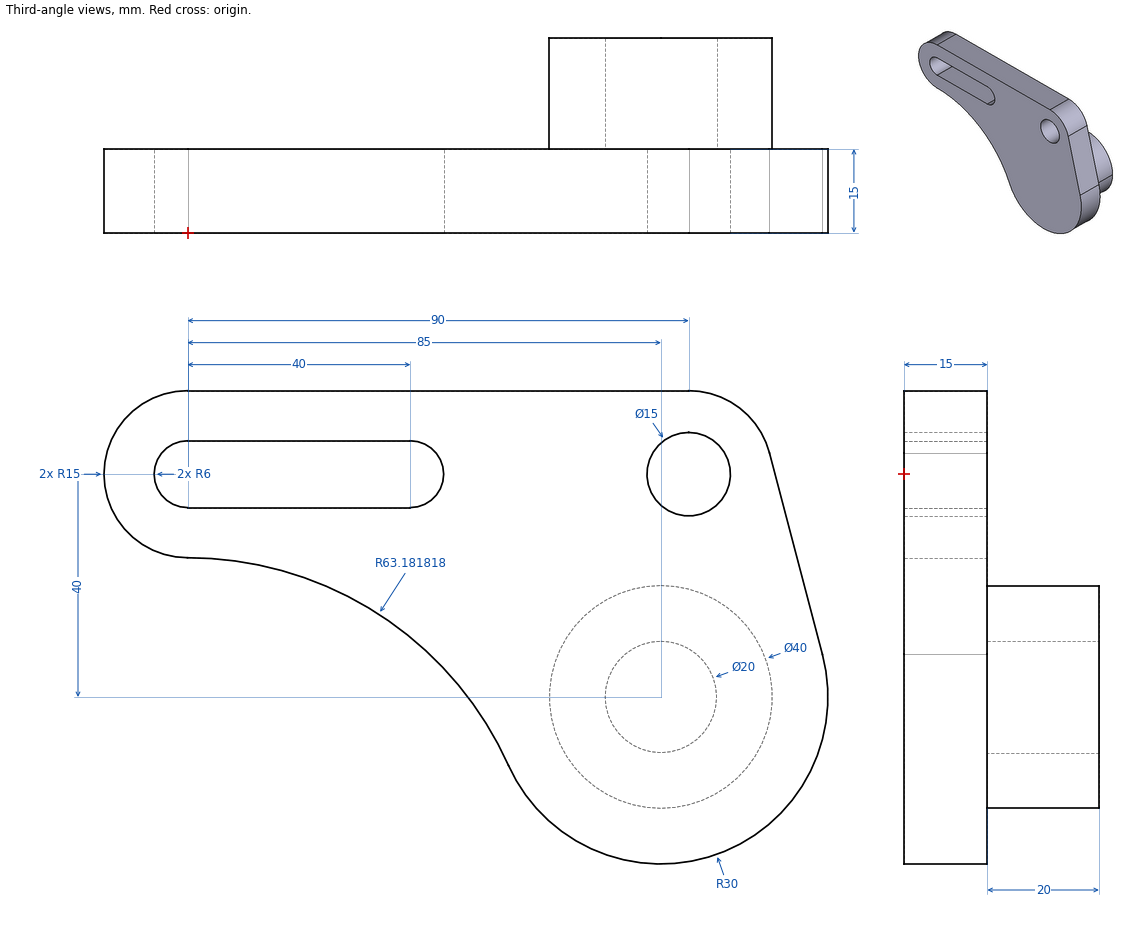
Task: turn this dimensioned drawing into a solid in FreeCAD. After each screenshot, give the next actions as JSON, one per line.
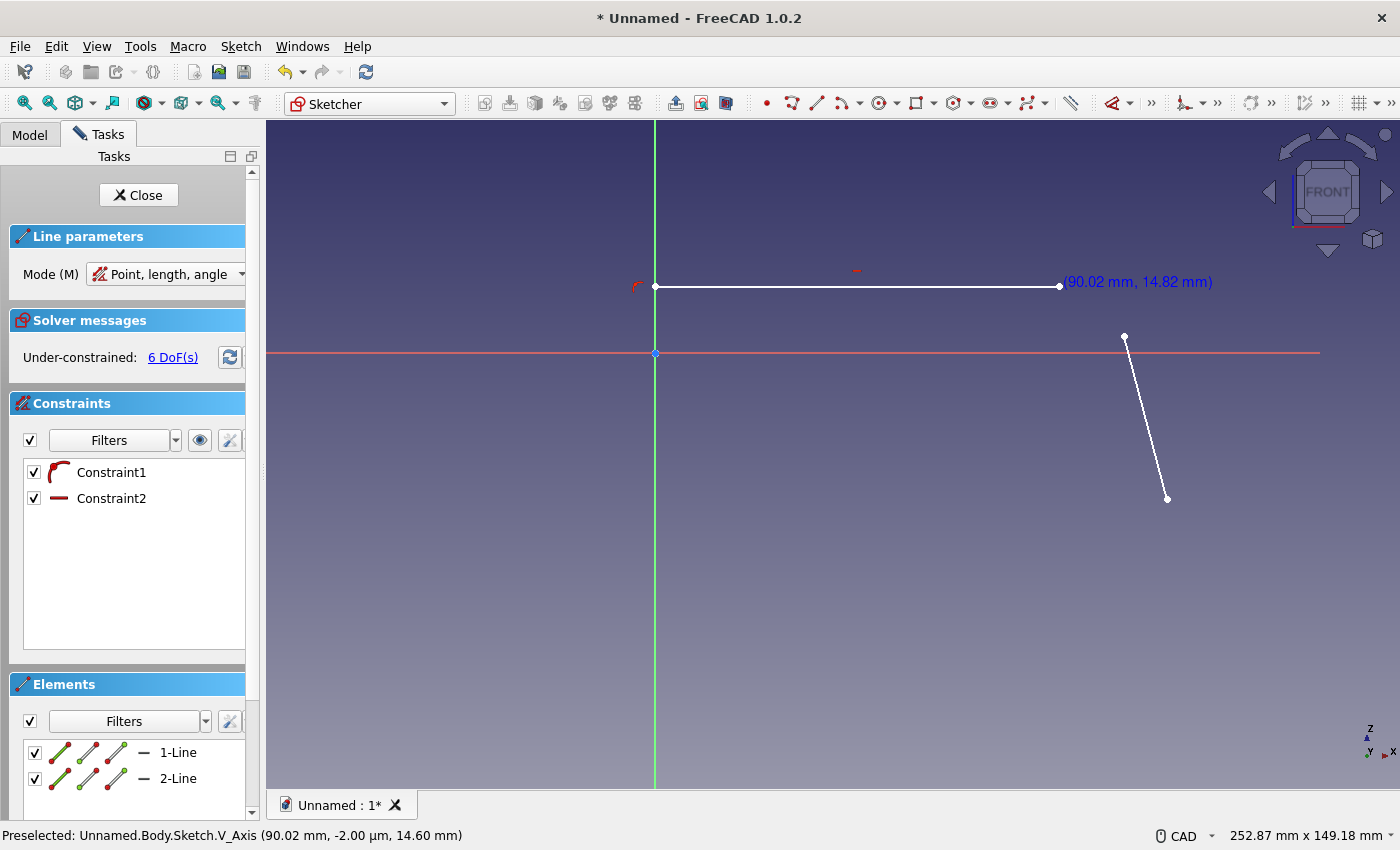
{"action": "left_click", "coordinate": [860, 104]}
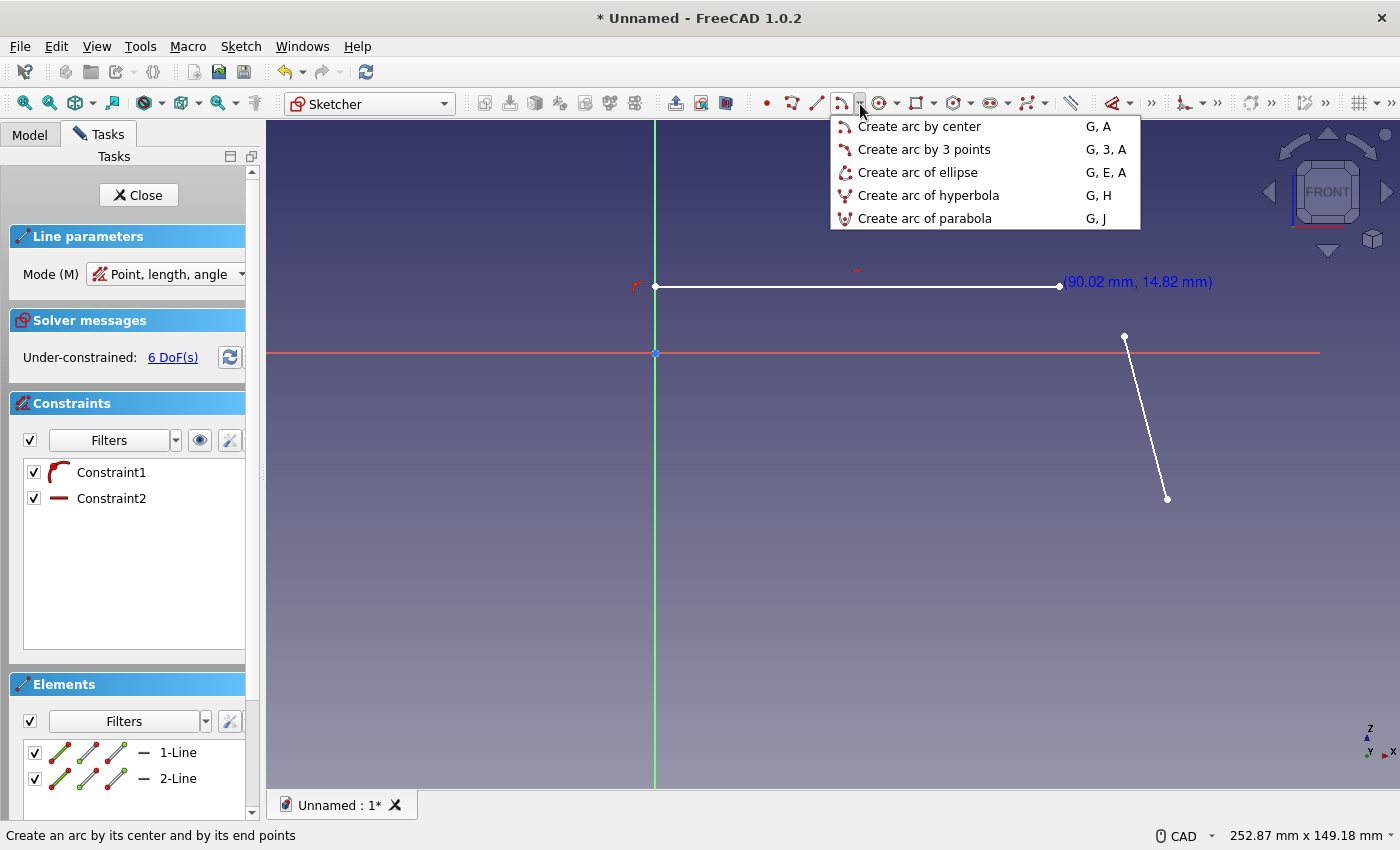
{"action": "left_click", "coordinate": [986, 150]}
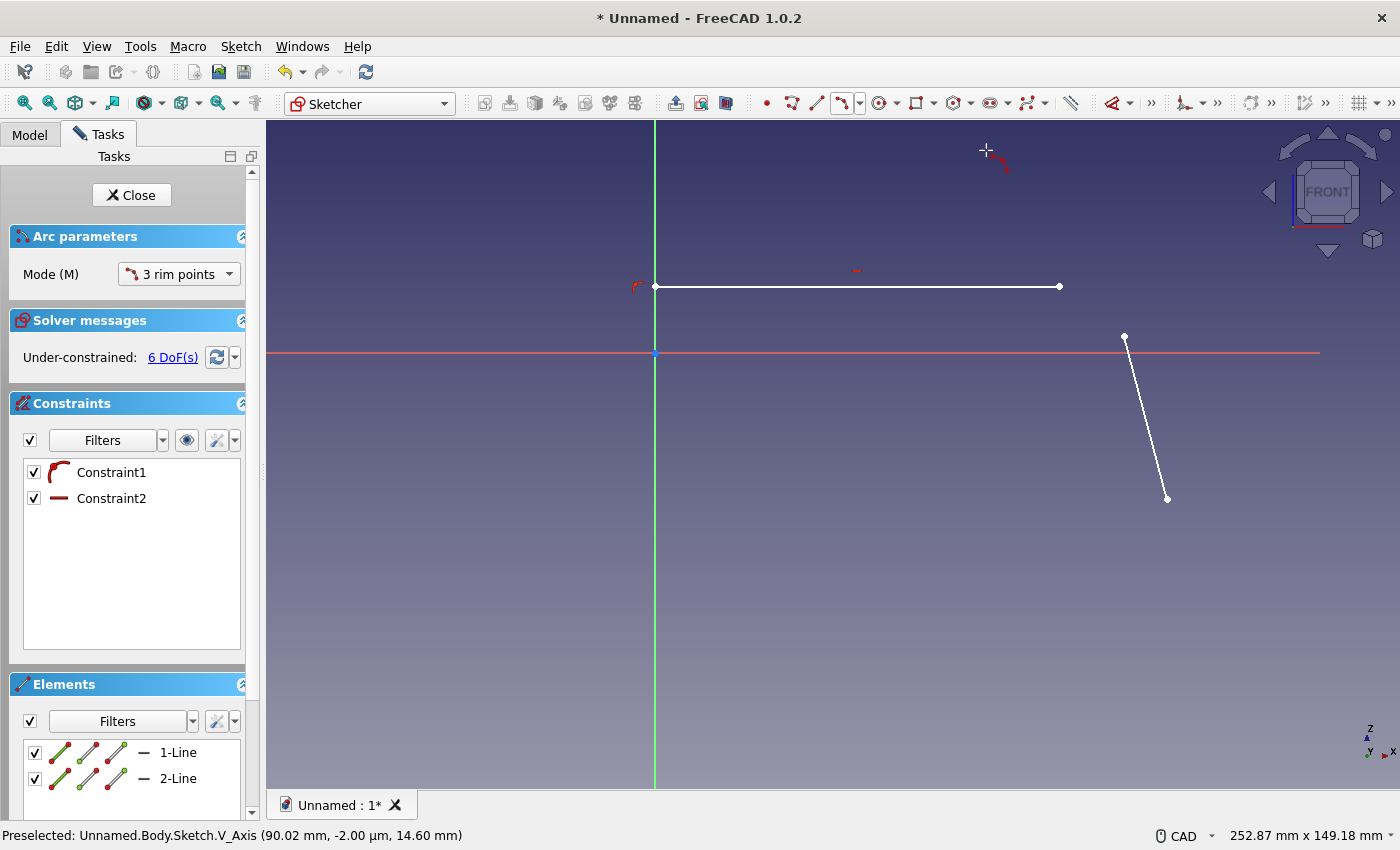
{"action": "left_click", "coordinate": [1167, 500]}
{"action": "left_click", "coordinate": [914, 588]}
{"action": "left_click", "coordinate": [1081, 660]}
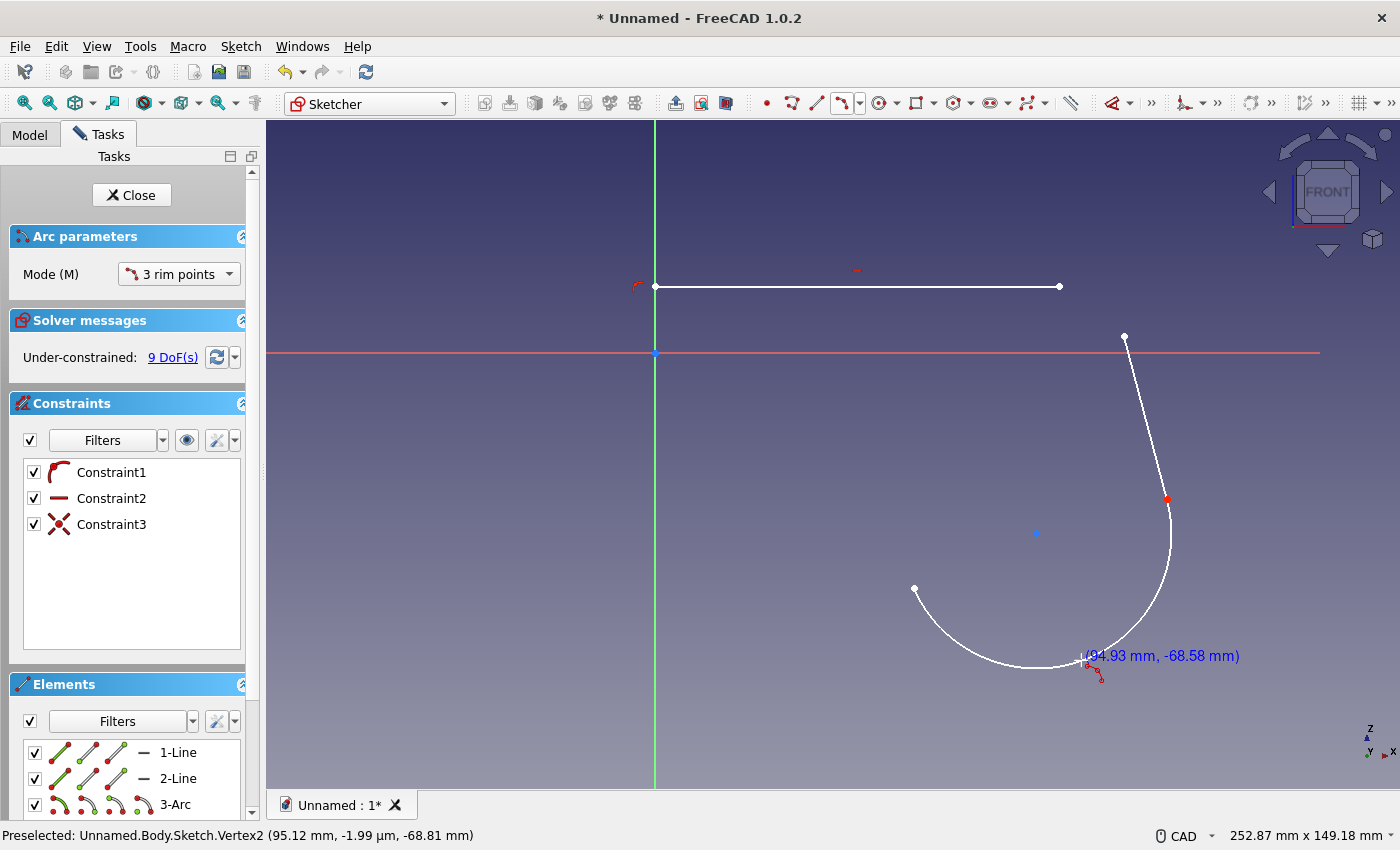
{"action": "left_click", "coordinate": [914, 589]}
{"action": "left_click", "coordinate": [655, 421]}
{"action": "left_click", "coordinate": [809, 466]}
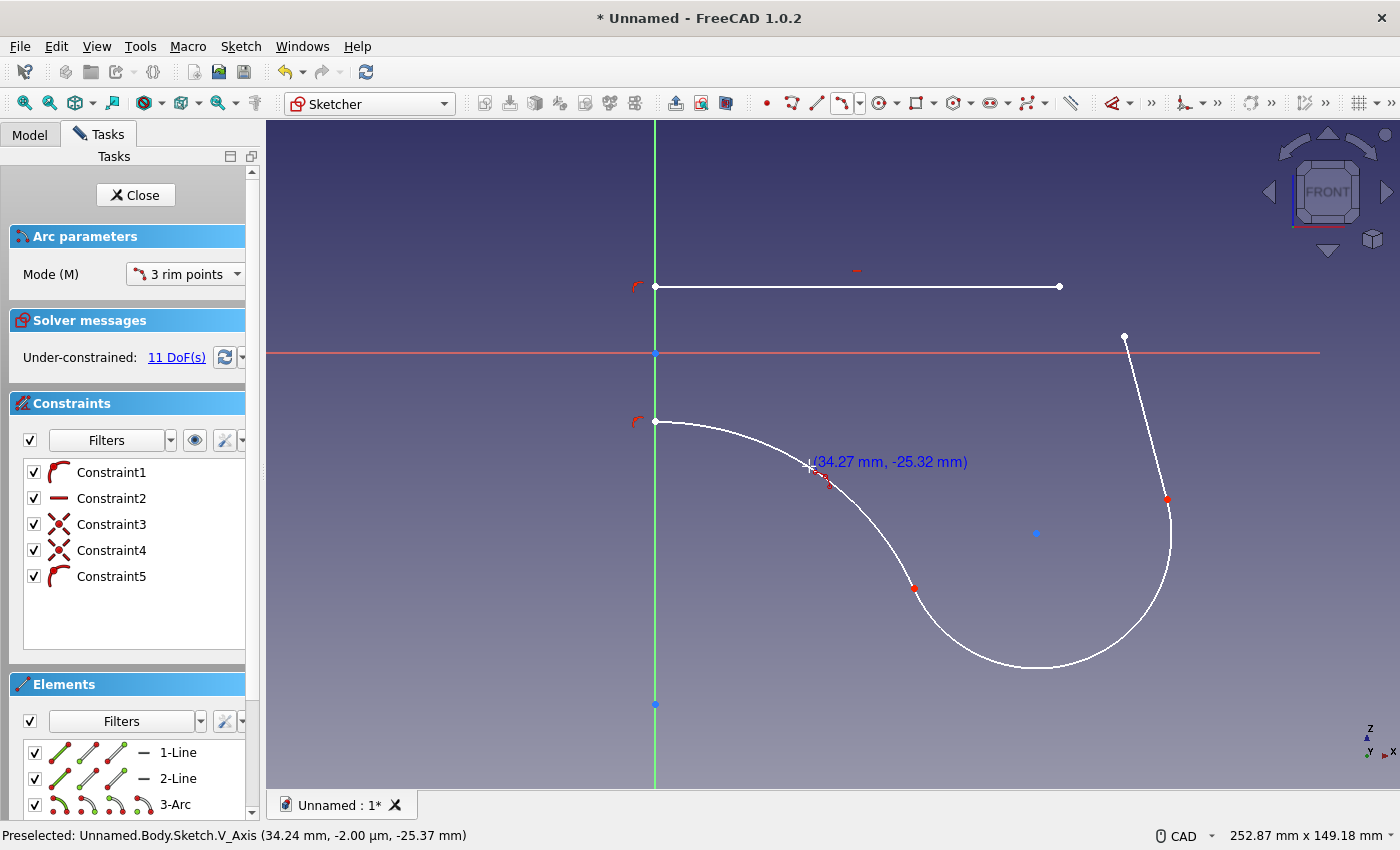
{"action": "left_click", "coordinate": [655, 422]}
{"action": "left_click", "coordinate": [655, 287]}
{"action": "left_click", "coordinate": [591, 333]}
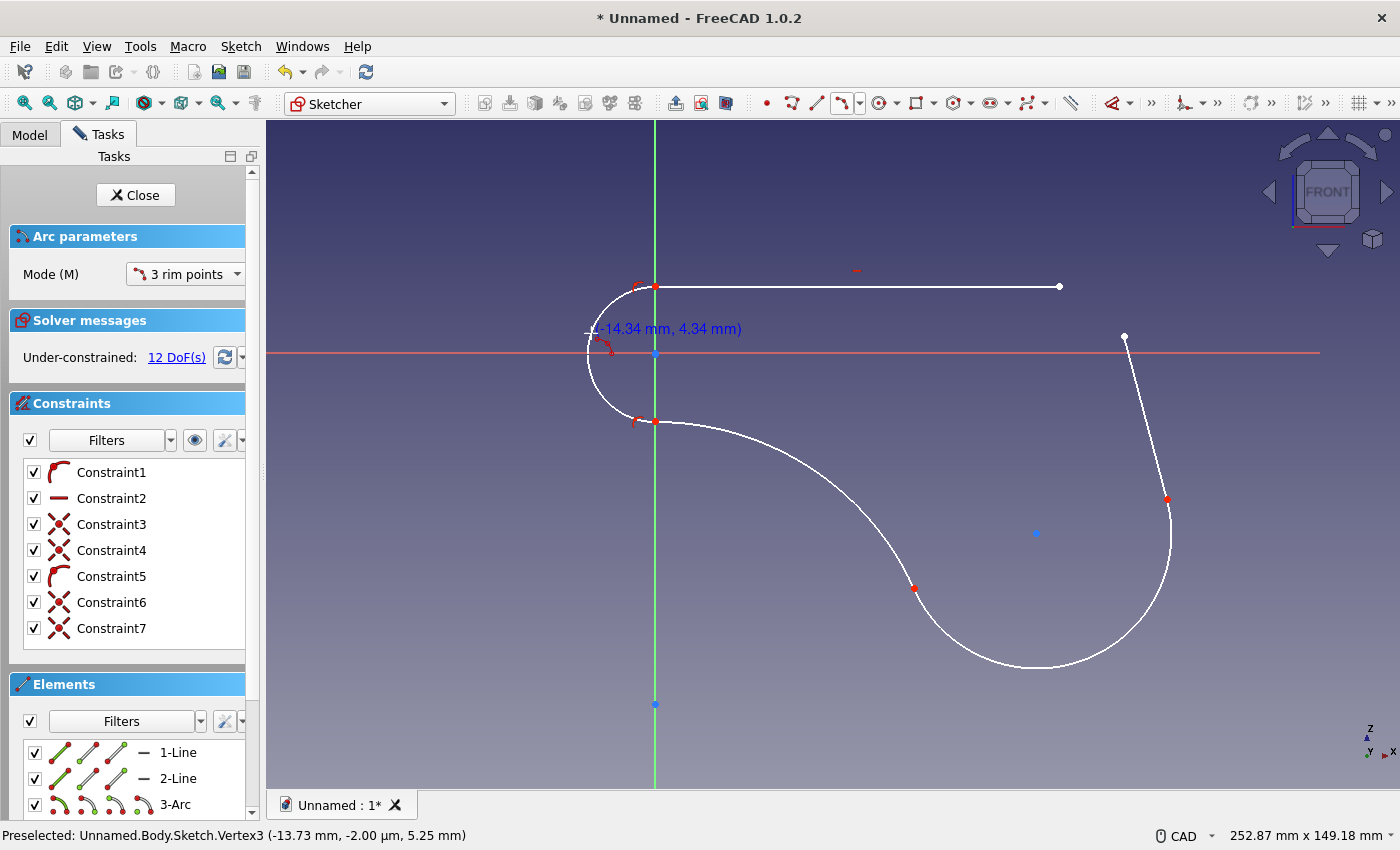
{"action": "left_click", "coordinate": [1059, 287]}
{"action": "left_click", "coordinate": [1124, 337]}
{"action": "left_click", "coordinate": [1100, 300]}
{"action": "key", "text": "Escape"}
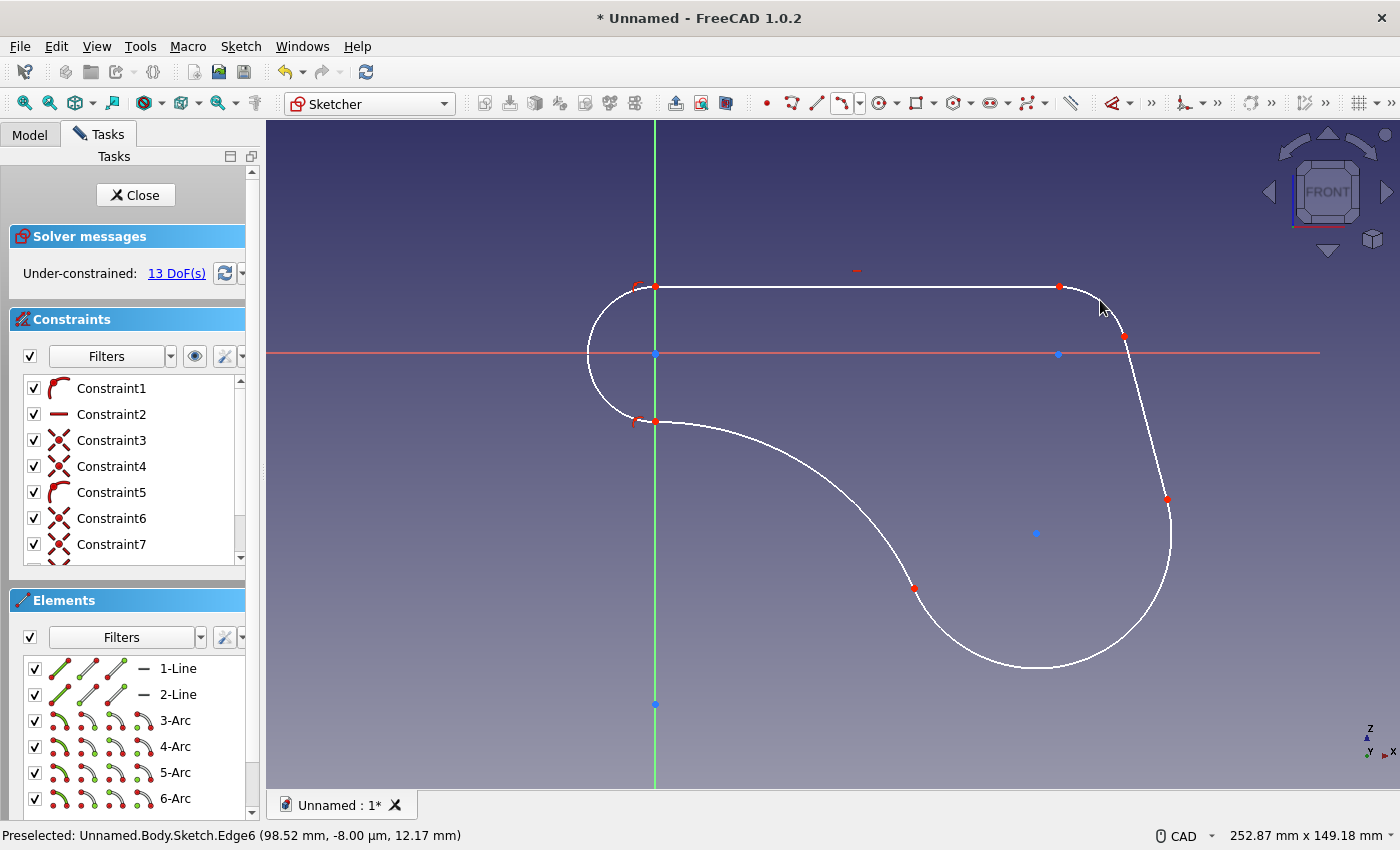
{"action": "left_click", "coordinate": [1137, 386]}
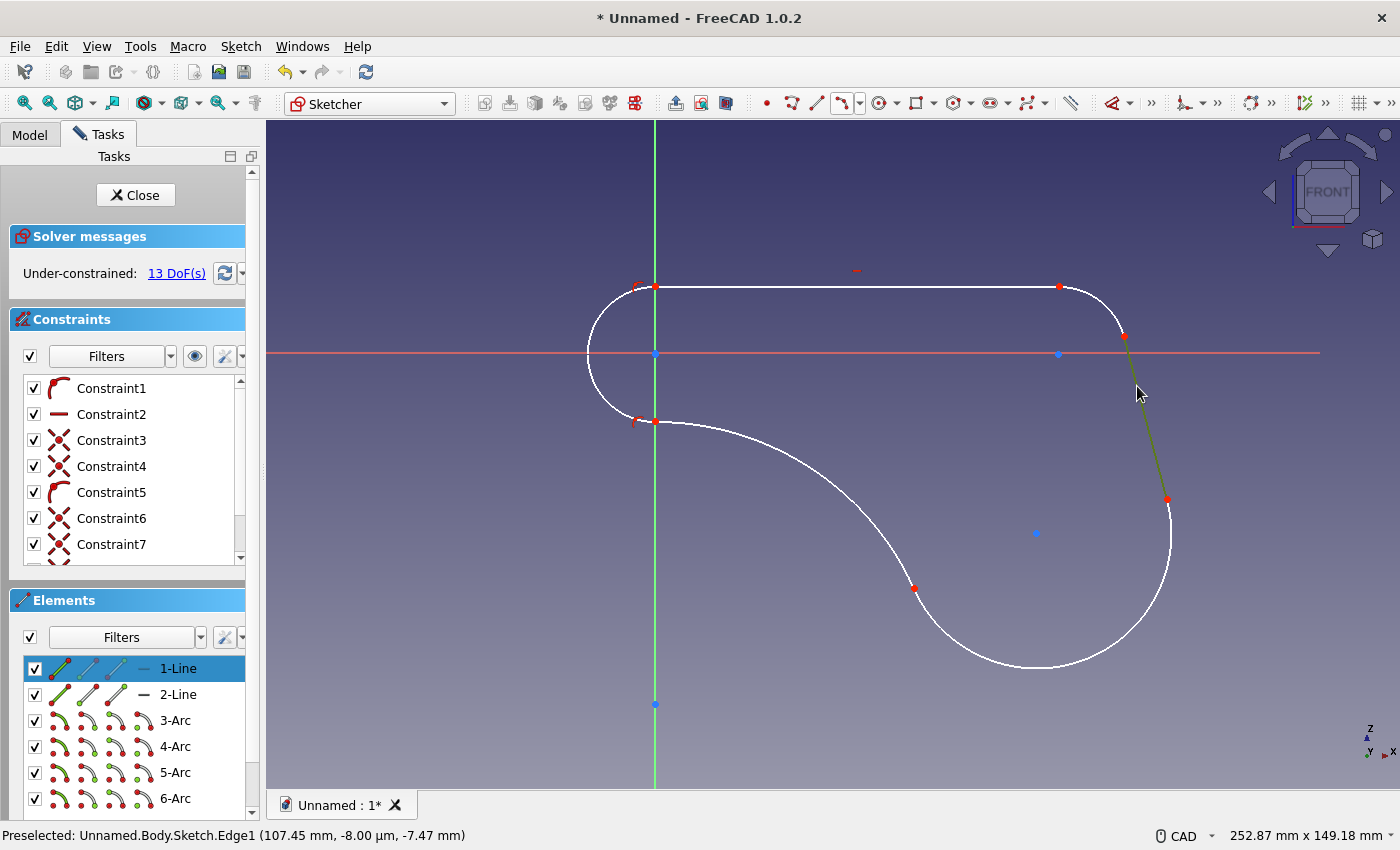
{"action": "left_click", "coordinate": [1003, 664]}